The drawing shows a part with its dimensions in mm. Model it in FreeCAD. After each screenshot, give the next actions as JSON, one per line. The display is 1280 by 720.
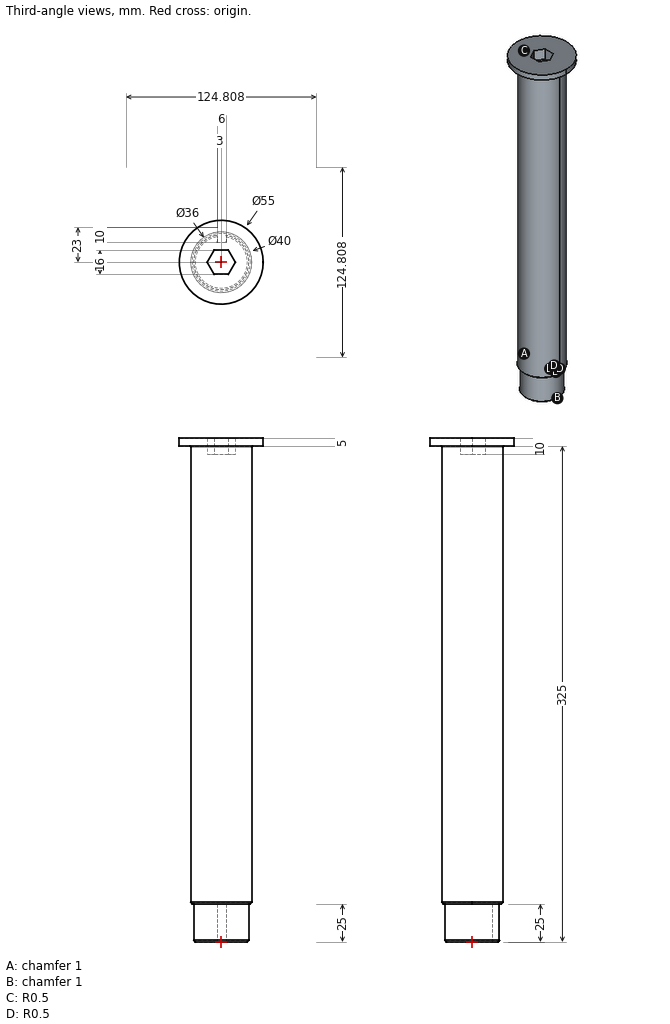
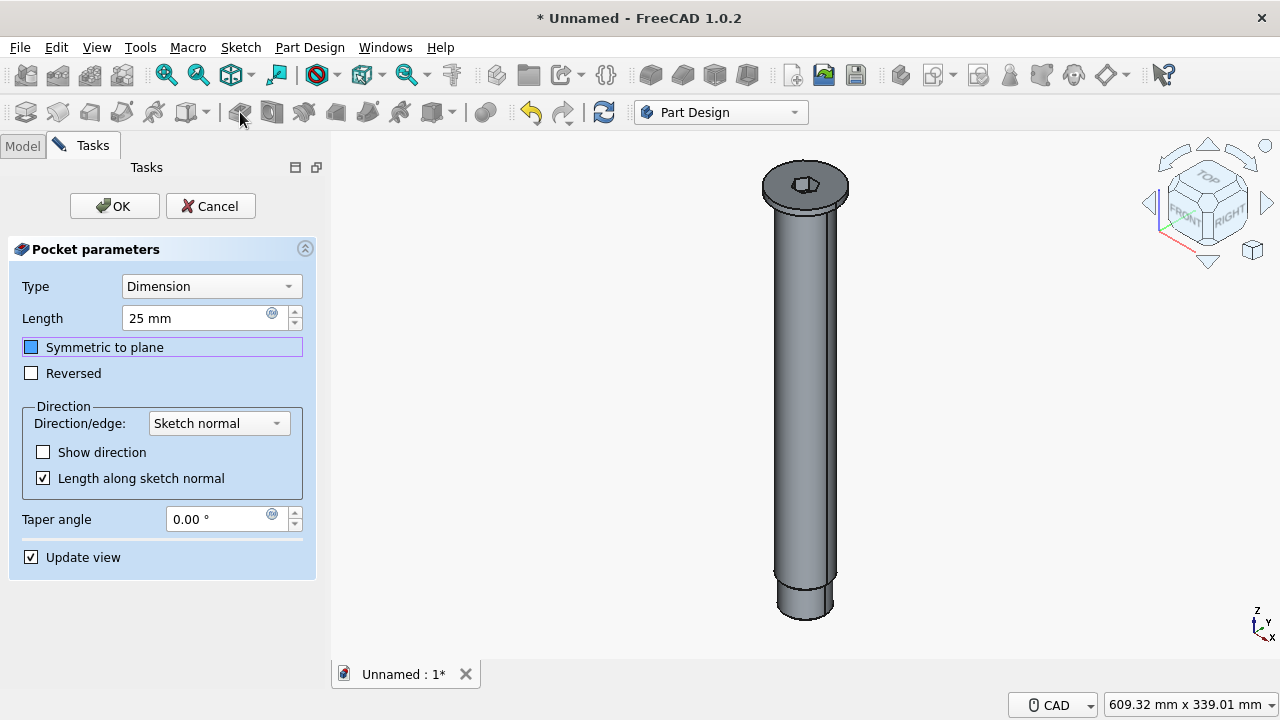
{"action": "left_click", "coordinate": [30, 373]}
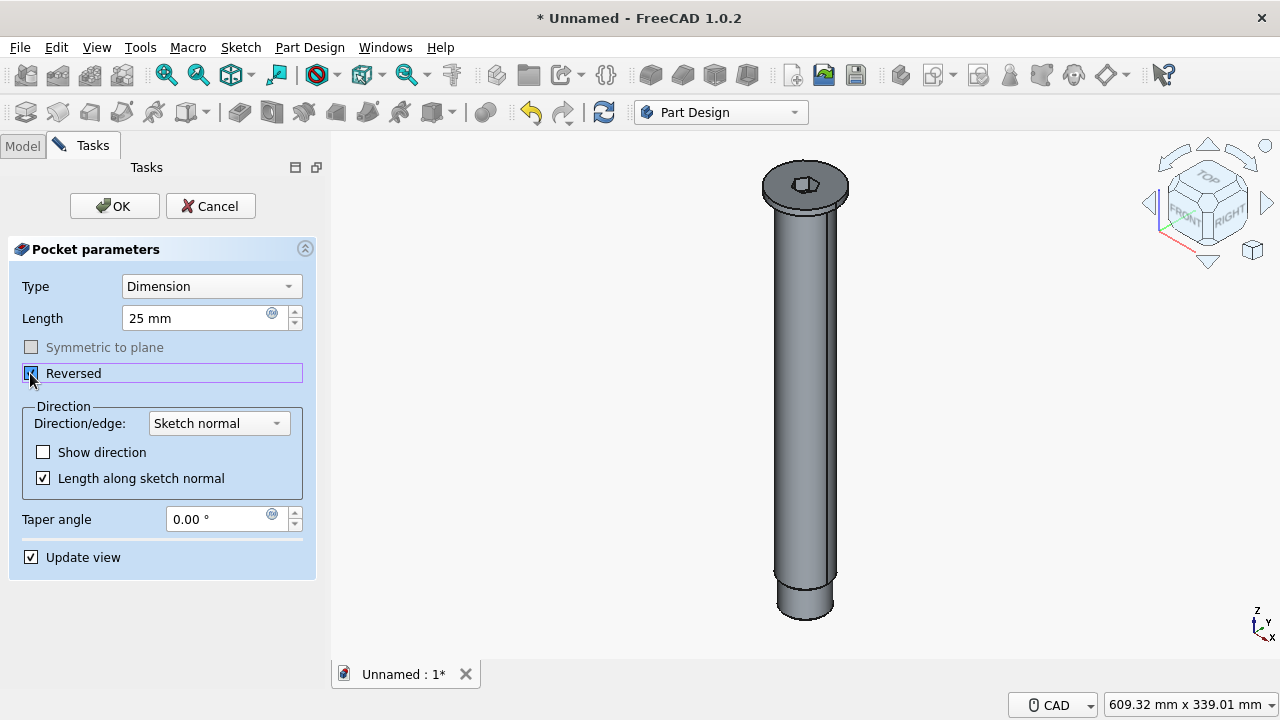
{"action": "left_click", "coordinate": [115, 206]}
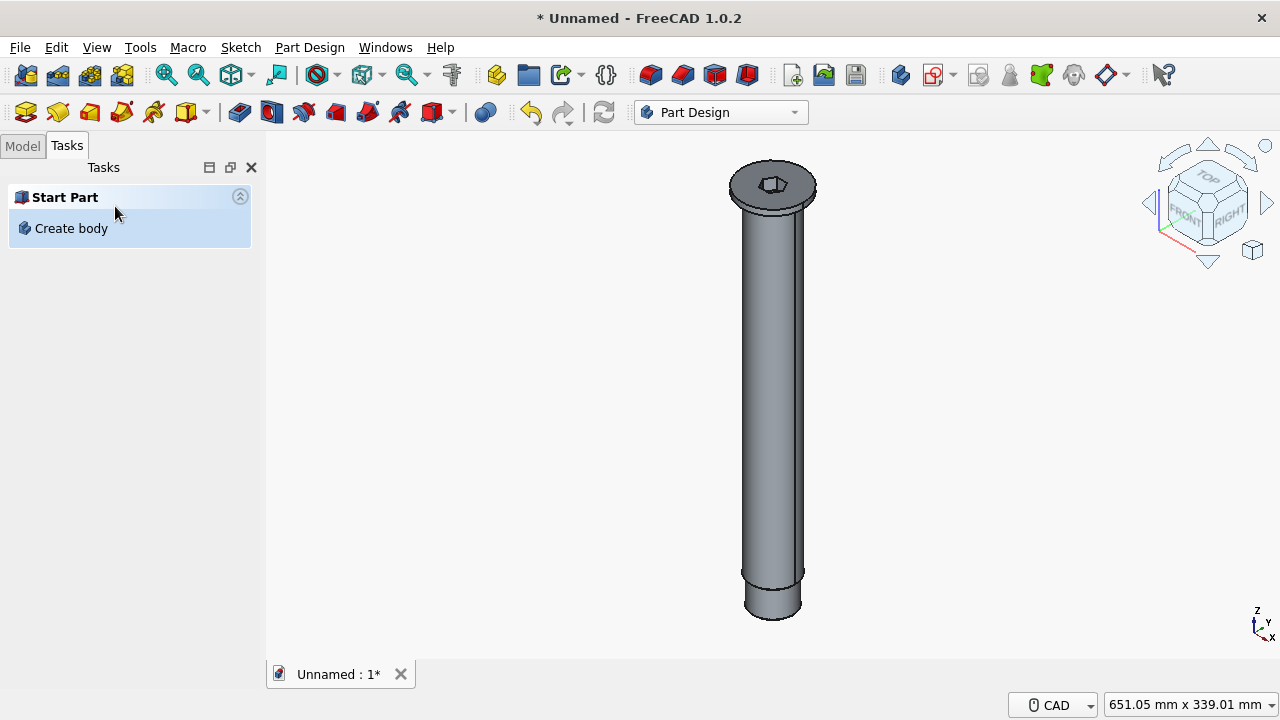
{"action": "key", "text": "2"}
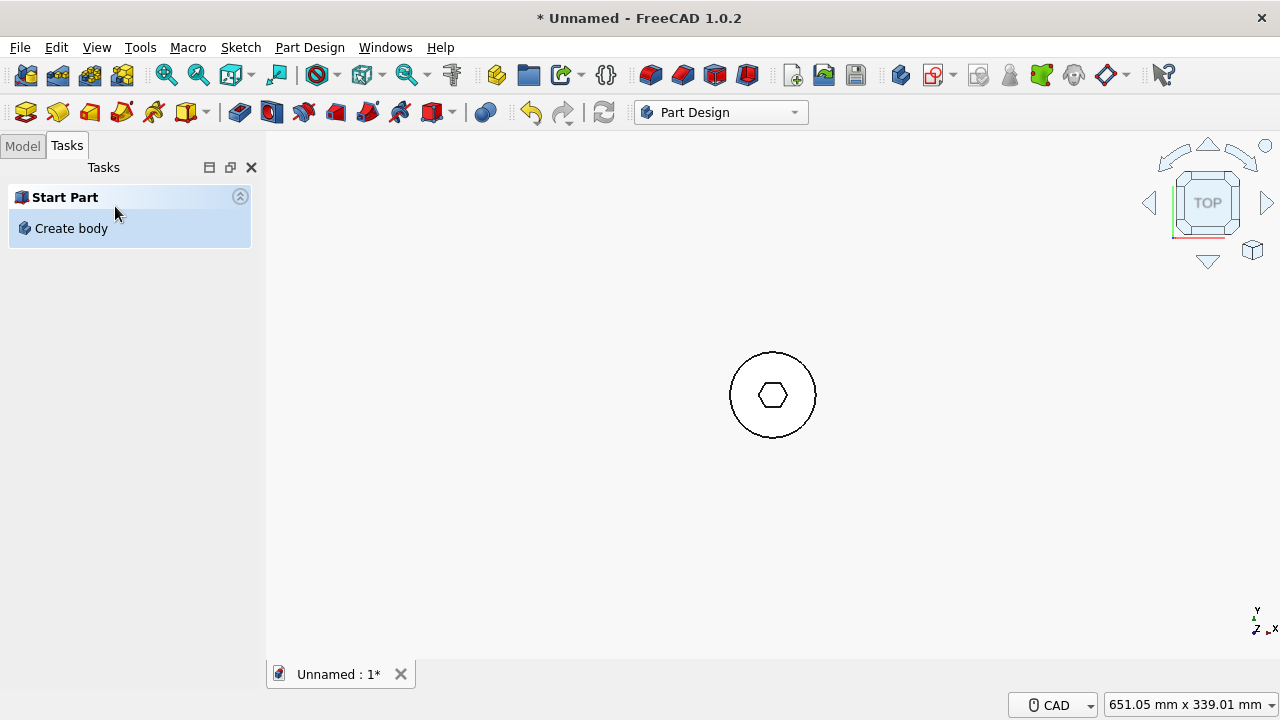
{"action": "left_click", "coordinate": [168, 76]}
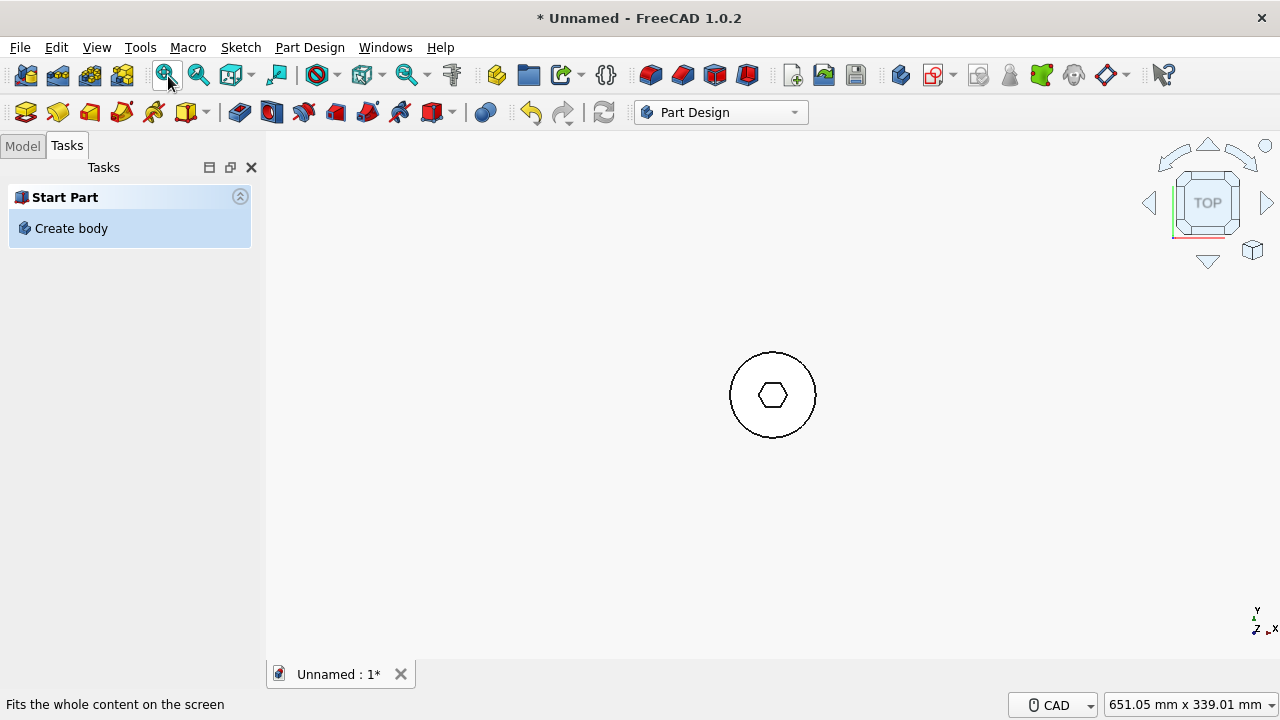
{"action": "key", "text": "0"}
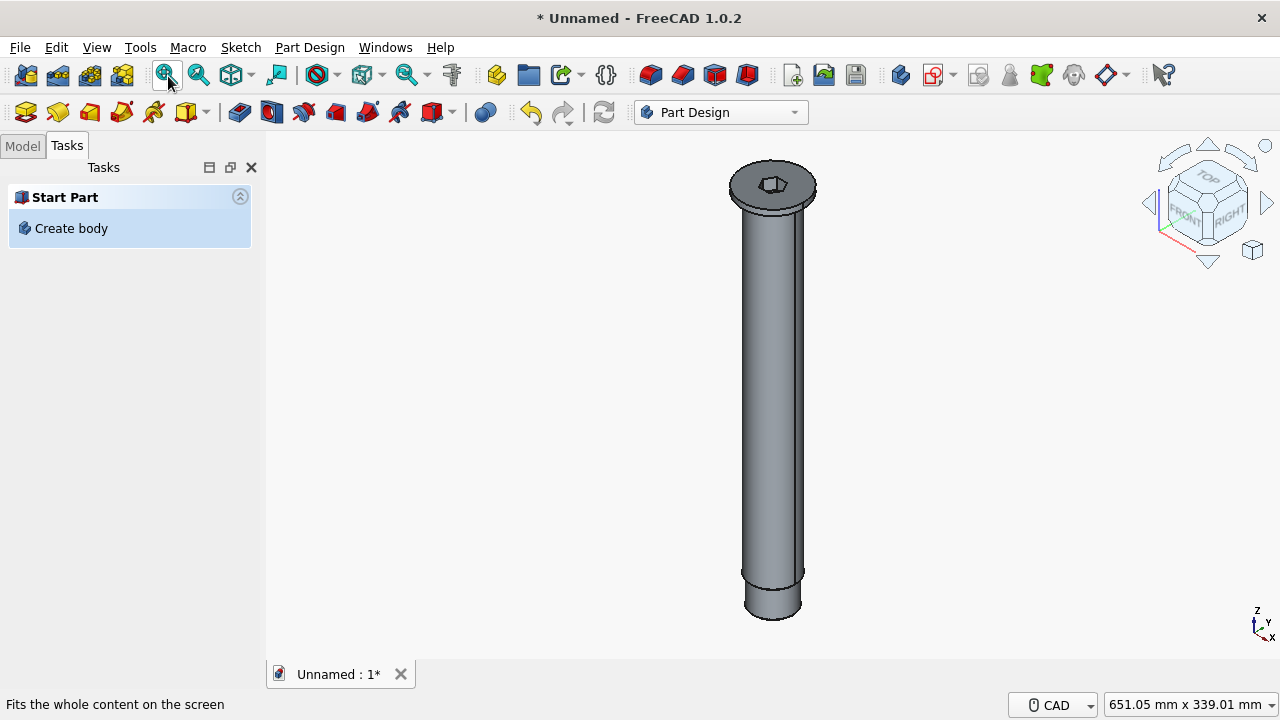
{"action": "key", "text": "1"}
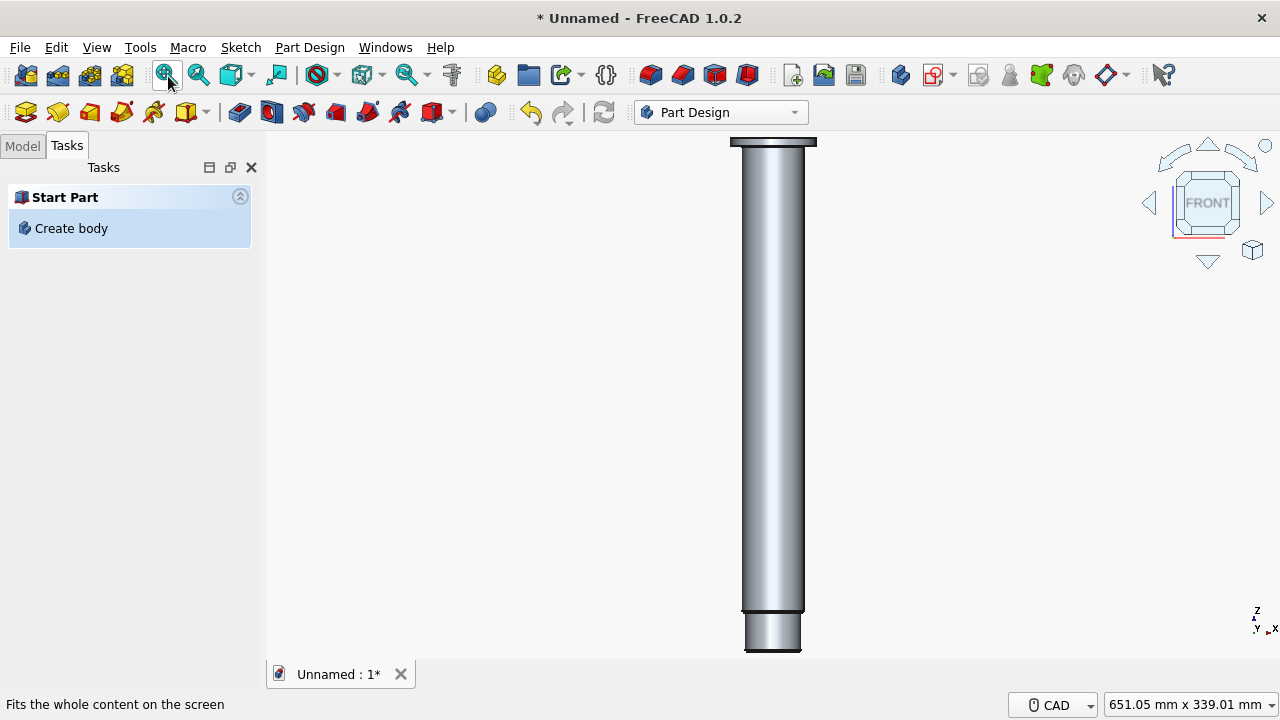
{"action": "key", "text": "3"}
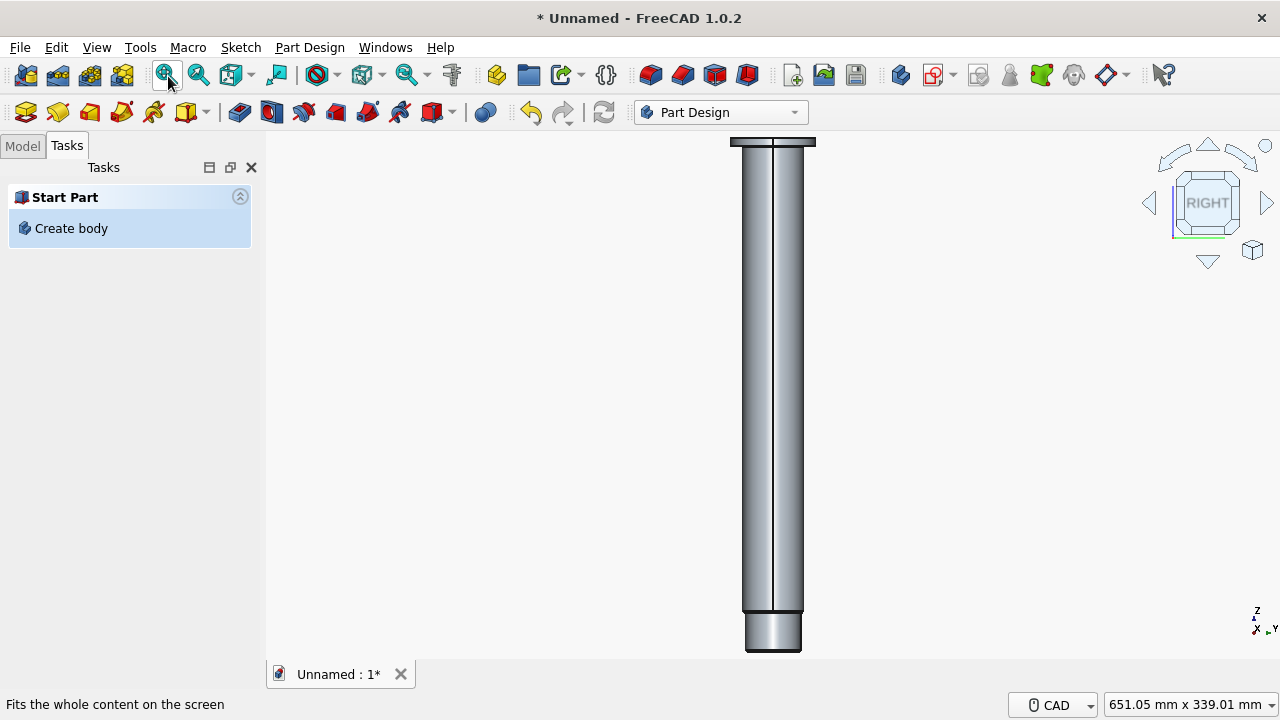
{"action": "key", "text": "5"}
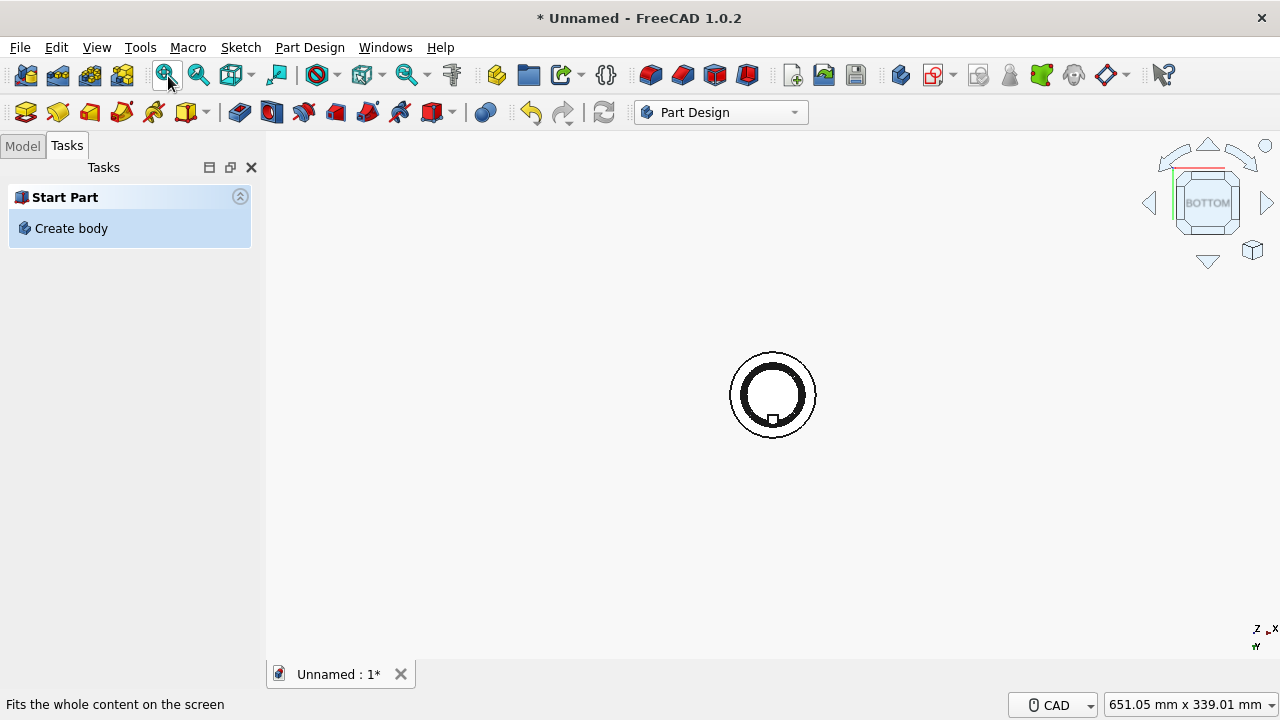
{"action": "left_click", "coordinate": [168, 76]}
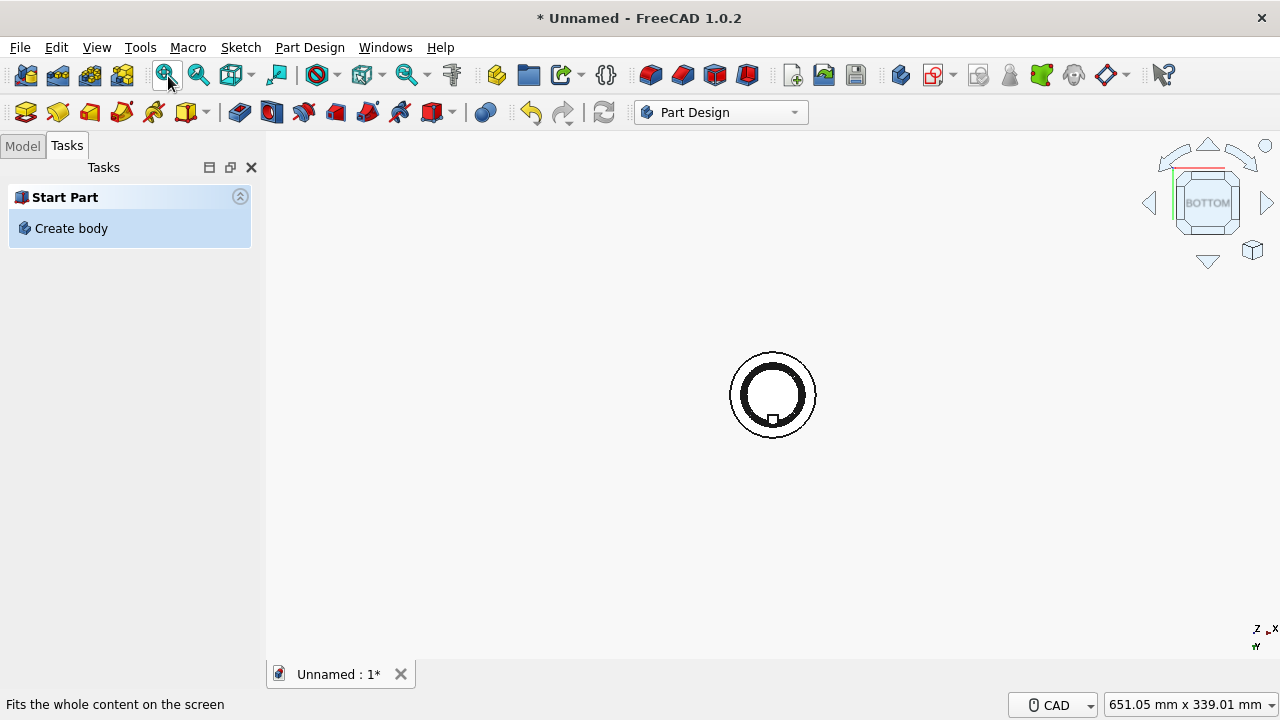
{"action": "key", "text": "4"}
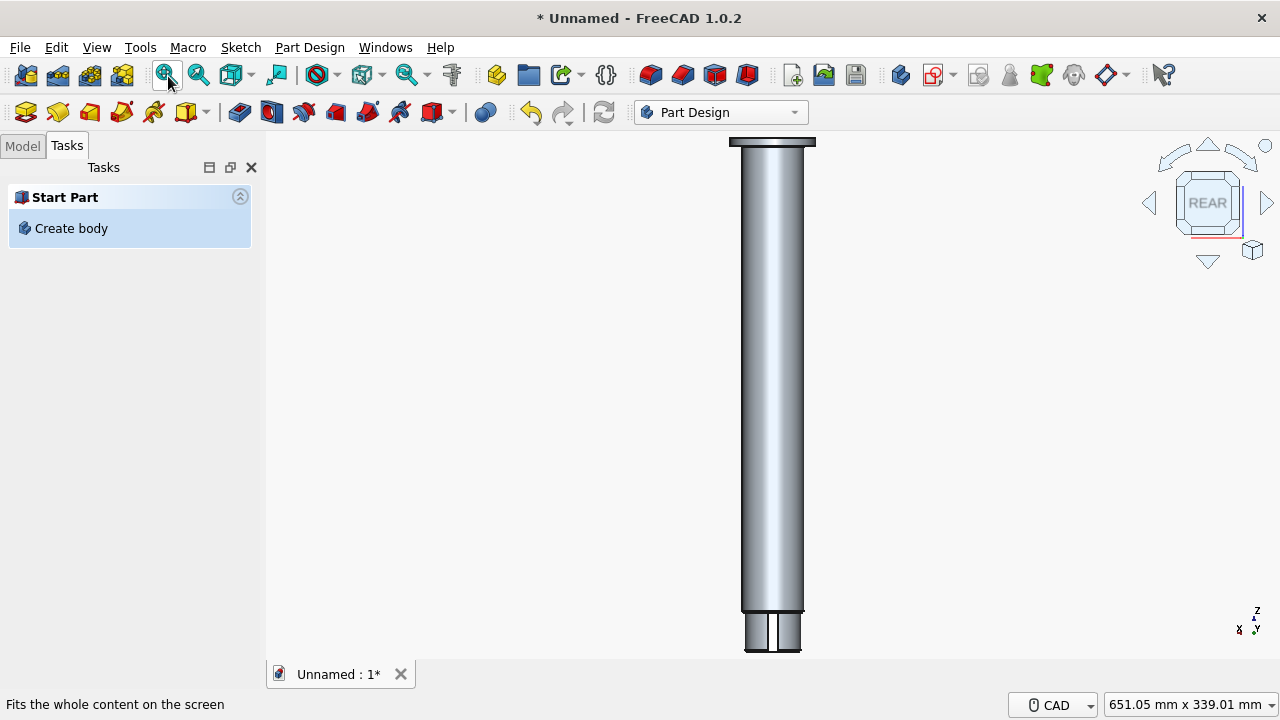
{"action": "left_click", "coordinate": [768, 627]}